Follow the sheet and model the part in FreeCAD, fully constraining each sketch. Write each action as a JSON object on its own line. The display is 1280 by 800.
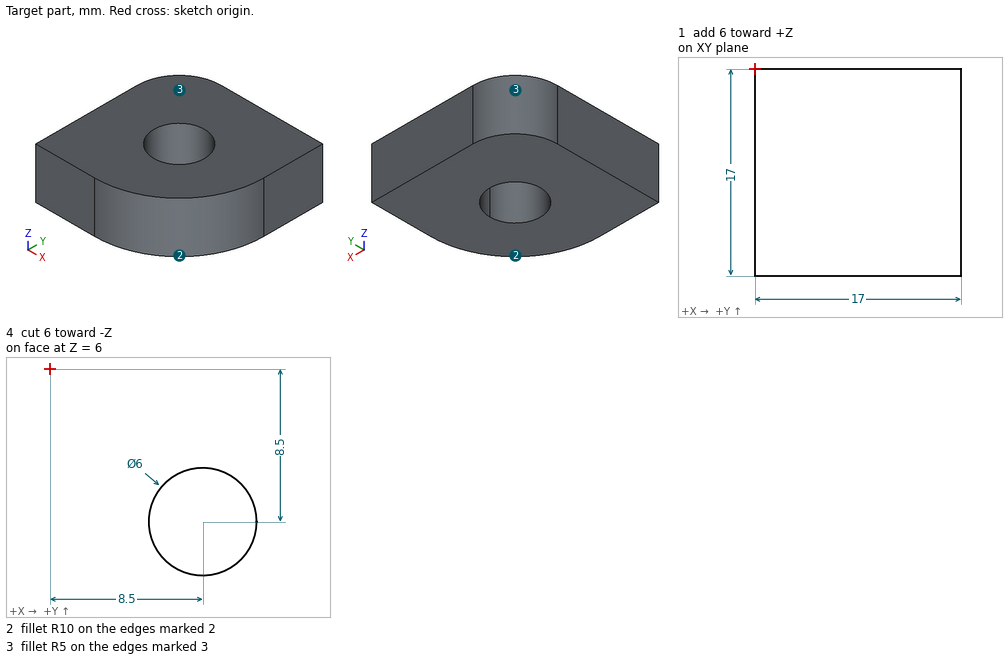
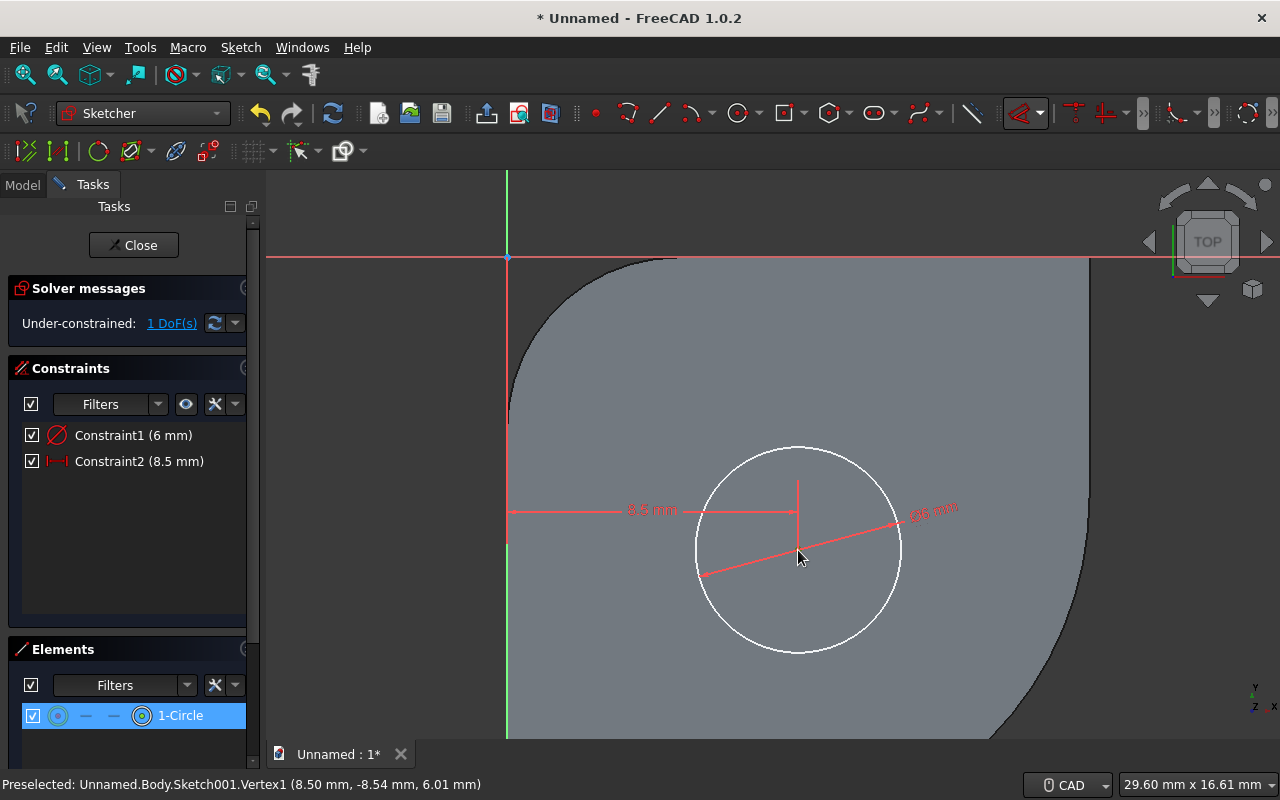
{"action": "left_click", "coordinate": [1042, 114]}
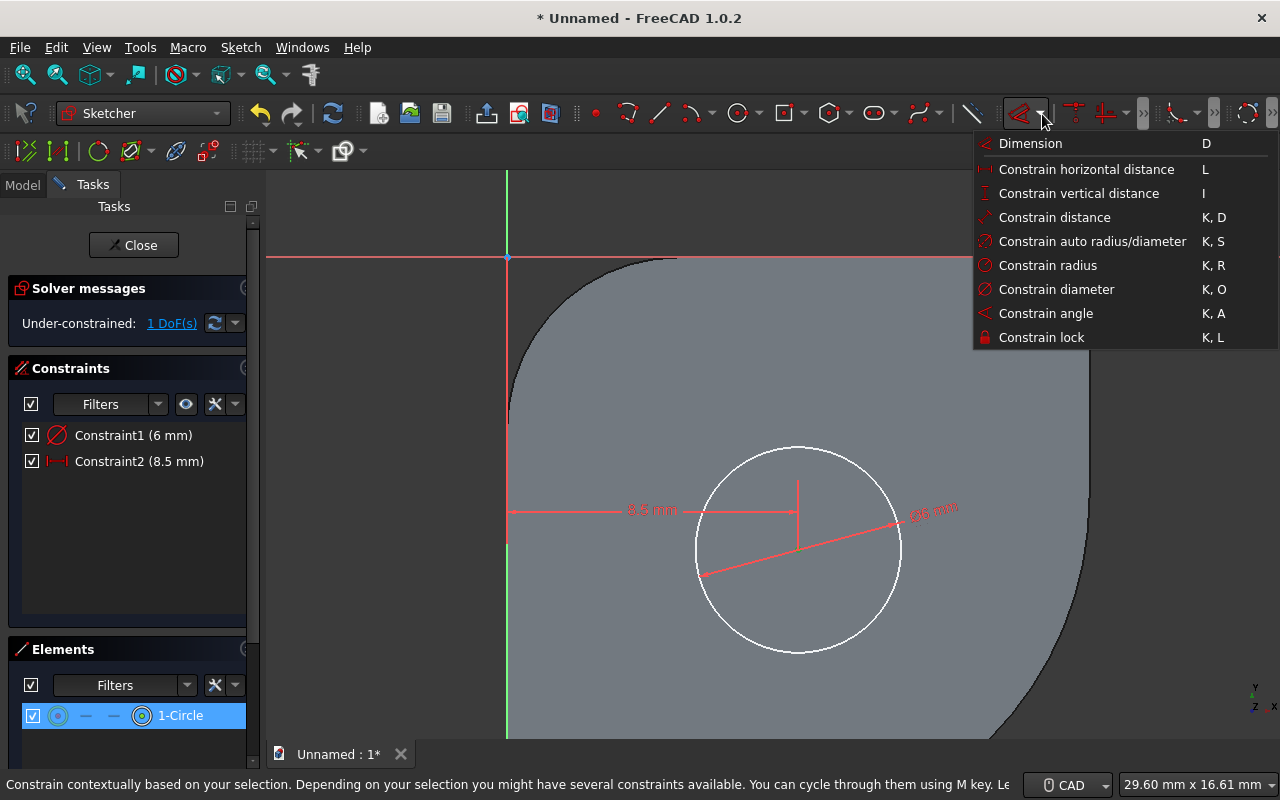
{"action": "left_click", "coordinate": [1126, 193]}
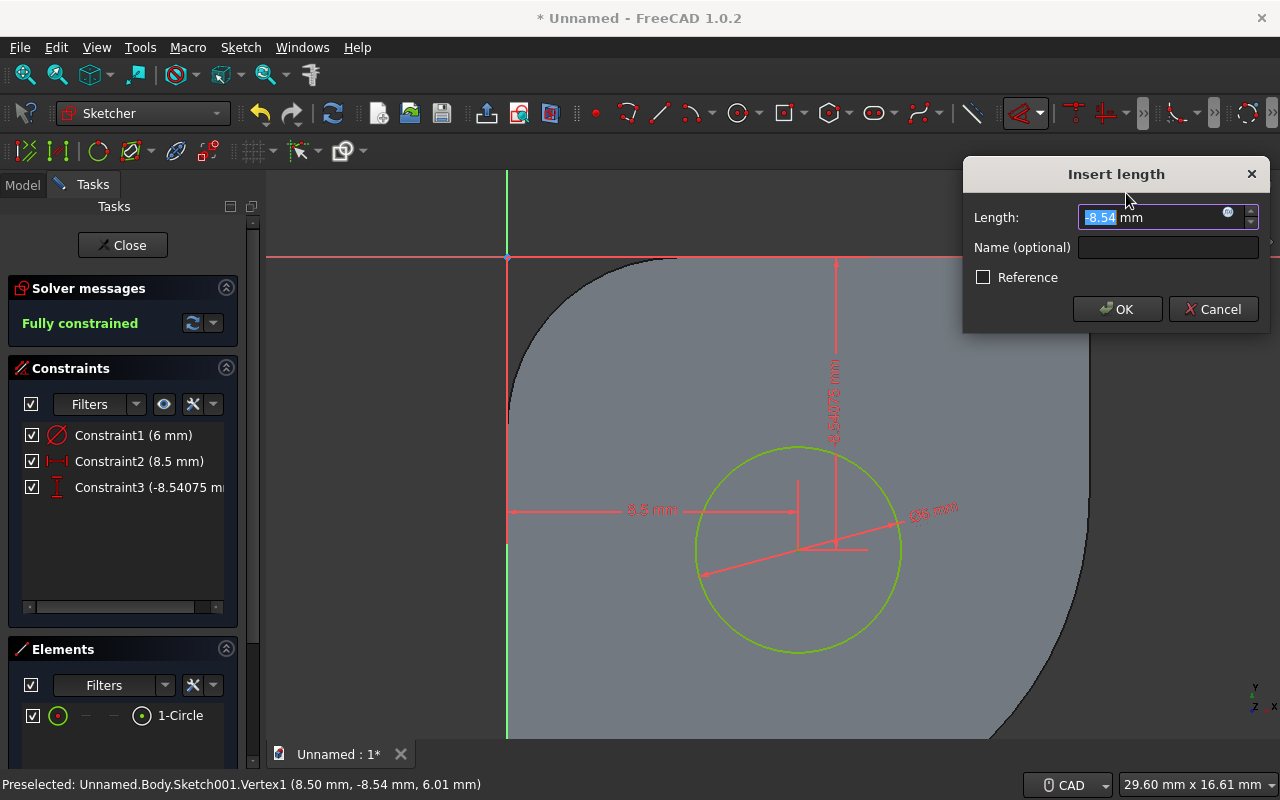
{"action": "type", "text": "-8.5"}
{"action": "key", "text": "Return"}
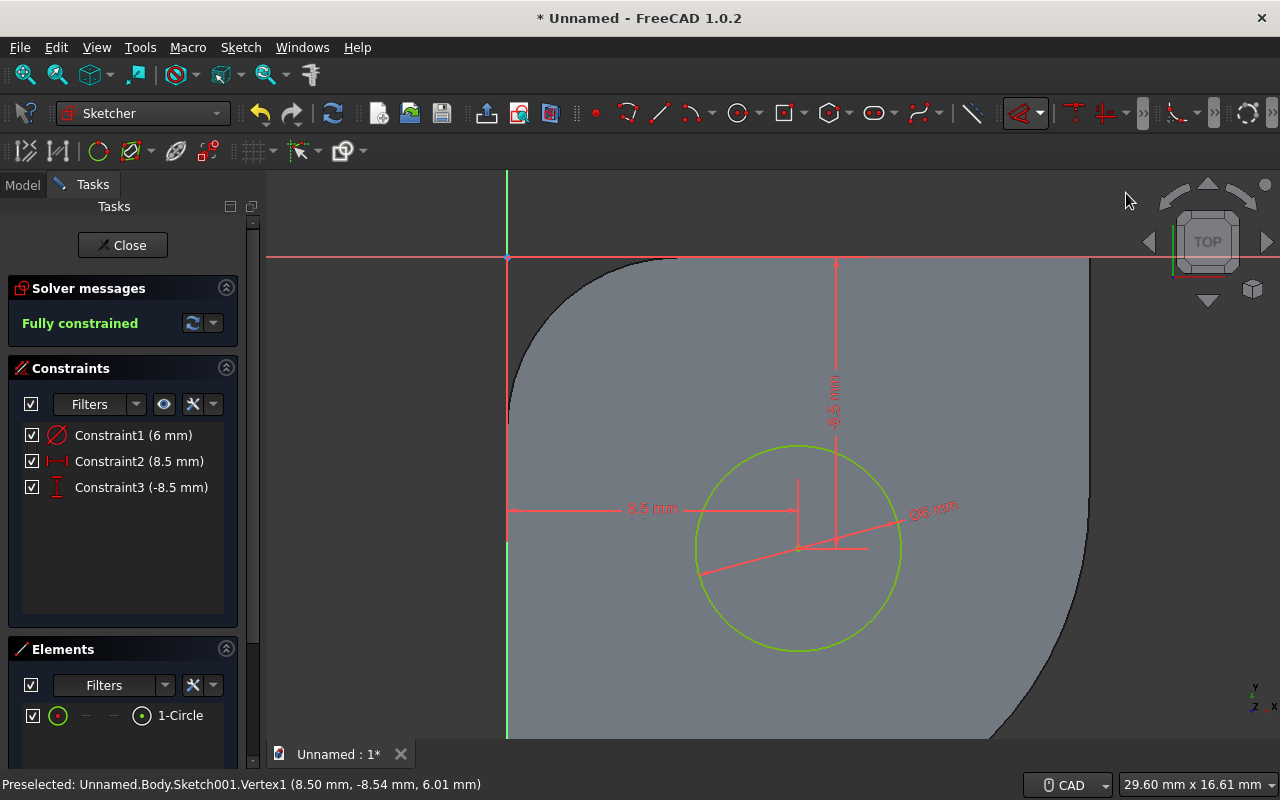
{"action": "left_click", "coordinate": [123, 245]}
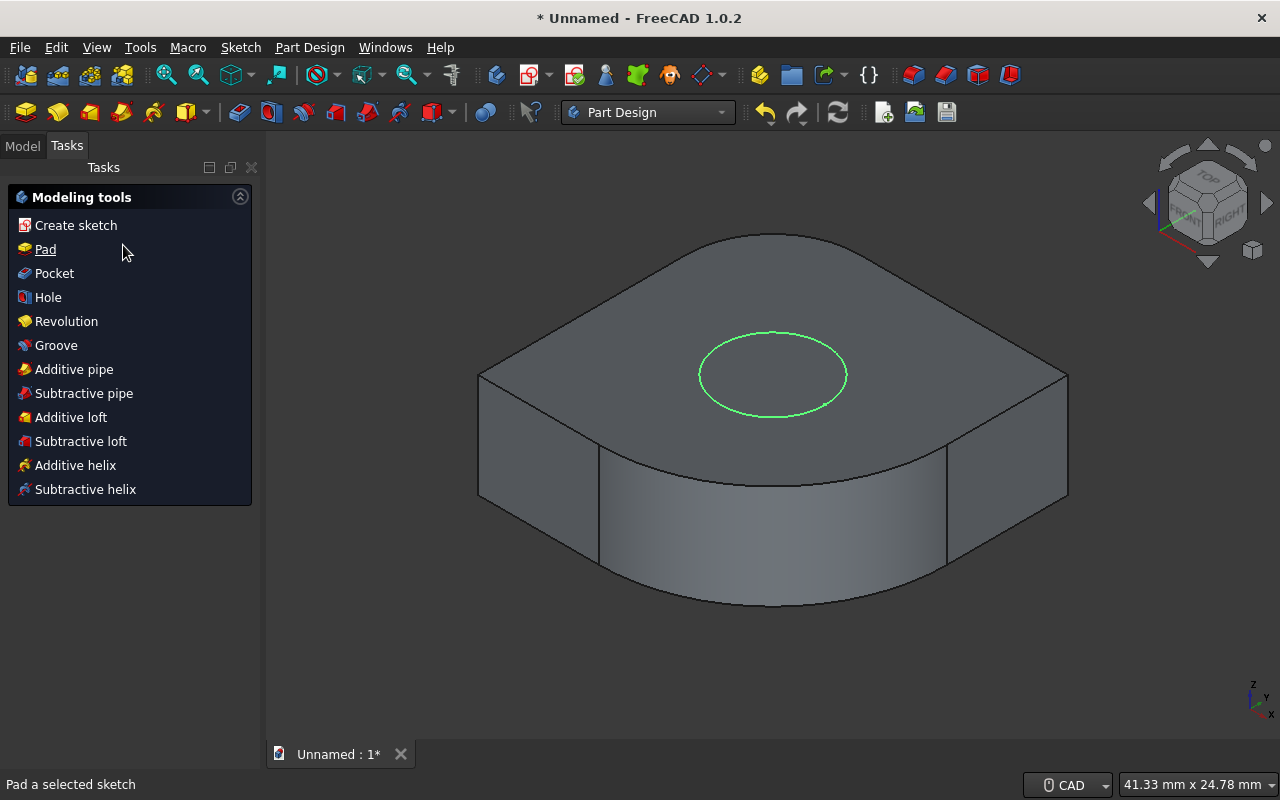
{"action": "left_click", "coordinate": [240, 112]}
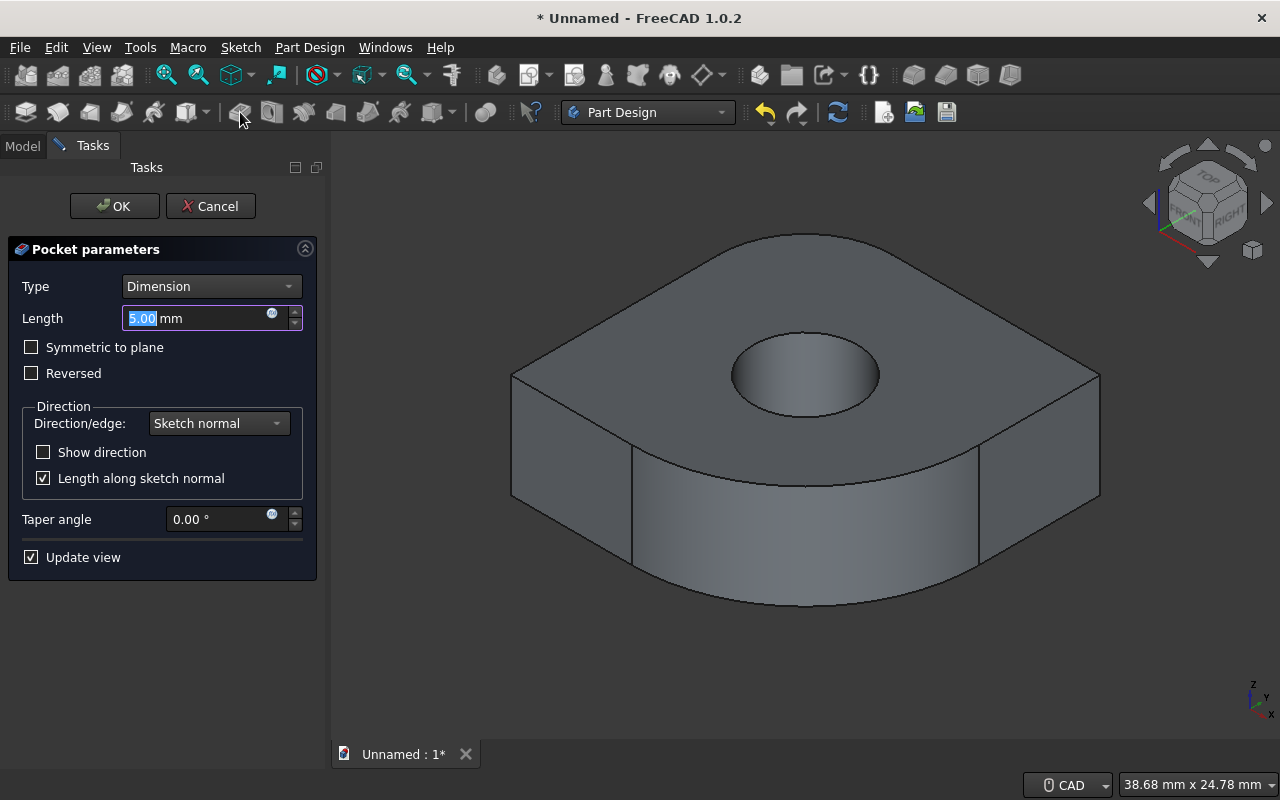
{"action": "type", "text": "6"}
{"action": "key", "text": "Tab"}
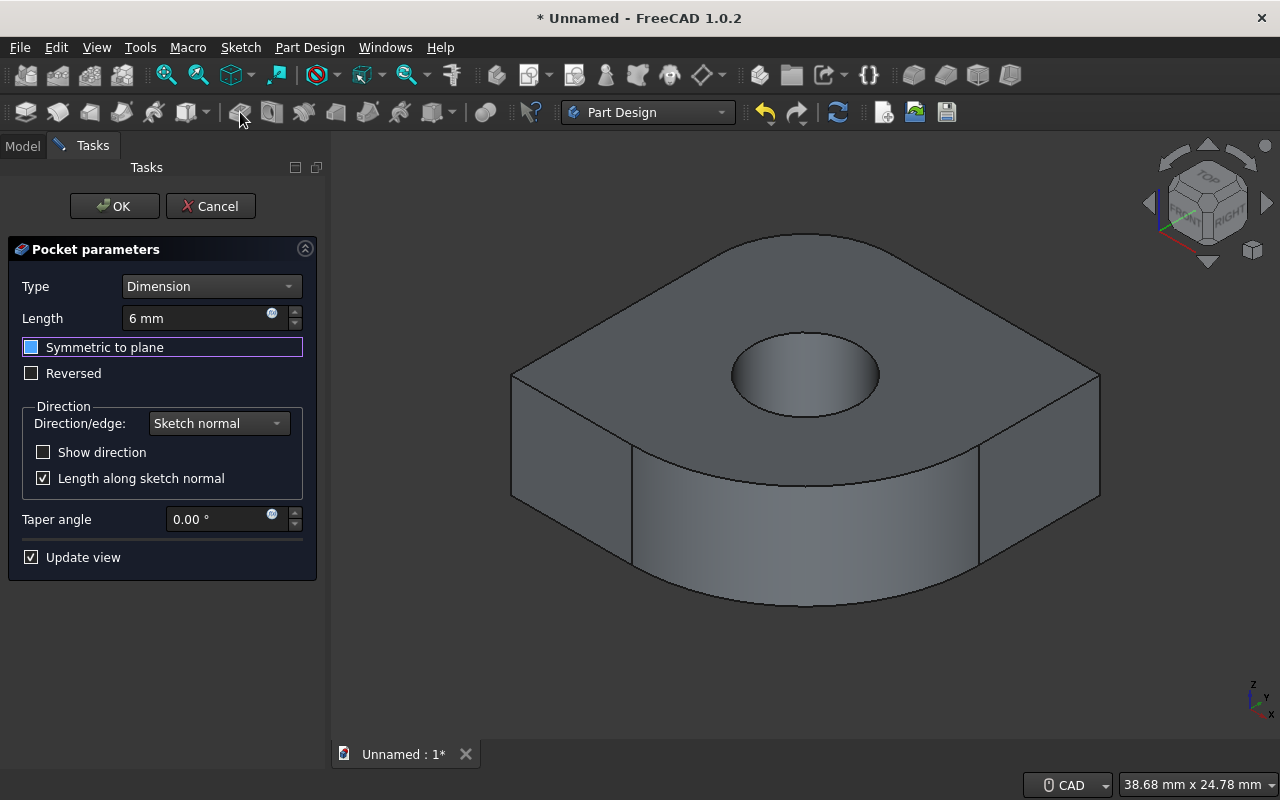
{"action": "left_click", "coordinate": [115, 206]}